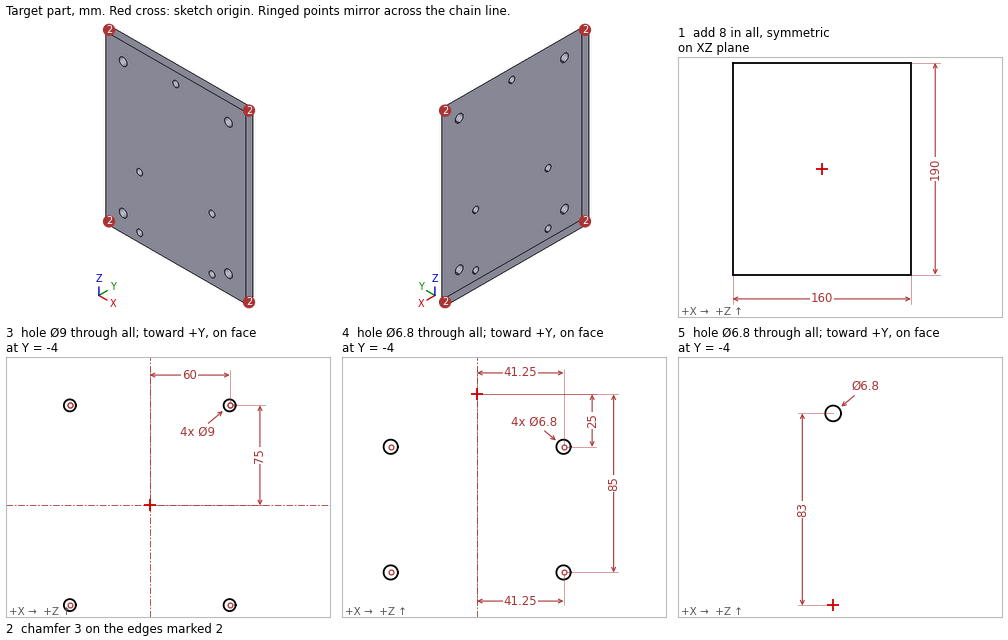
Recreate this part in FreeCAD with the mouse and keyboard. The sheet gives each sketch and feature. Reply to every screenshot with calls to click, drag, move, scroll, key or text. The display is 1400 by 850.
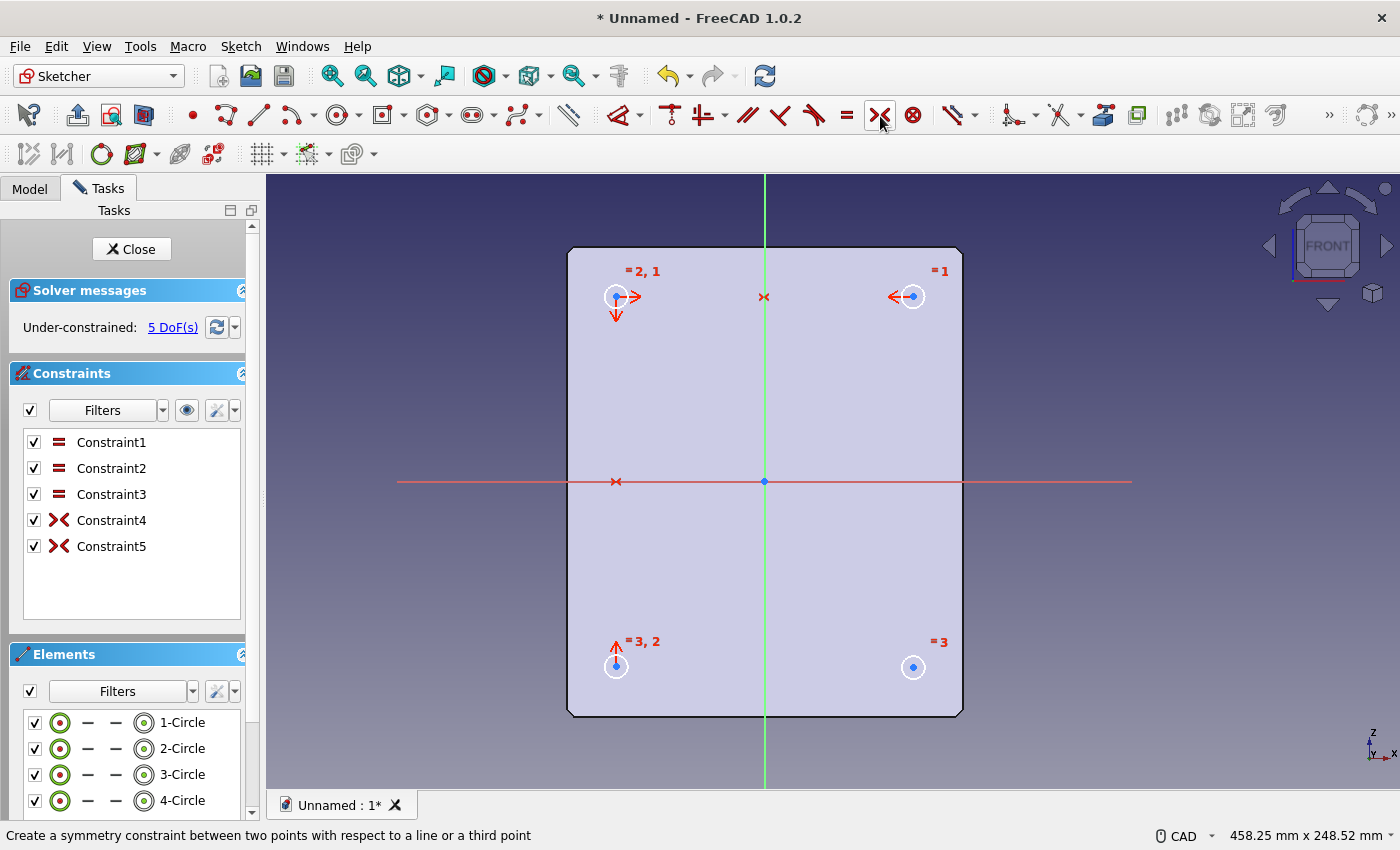
click(913, 297)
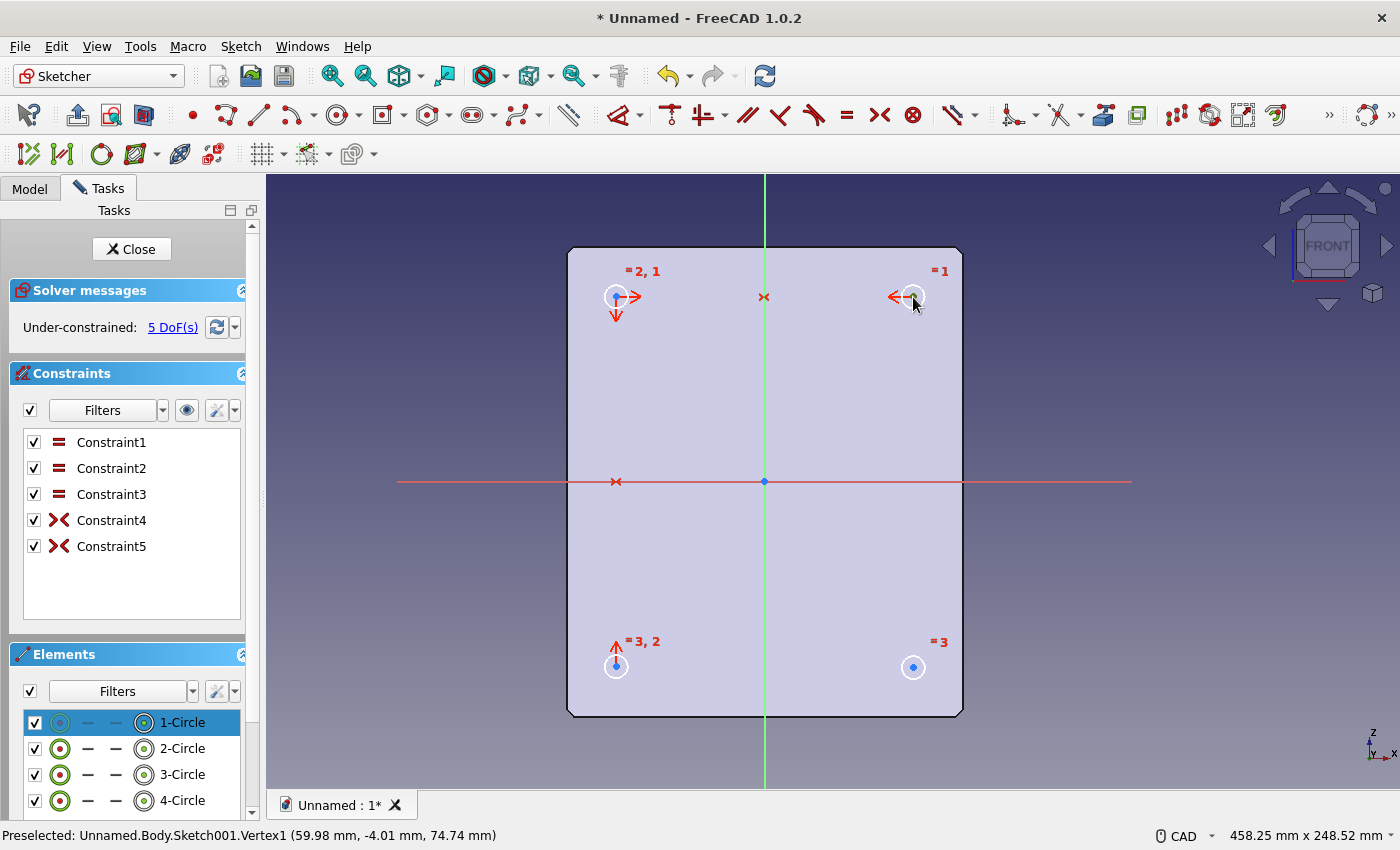
click(913, 668)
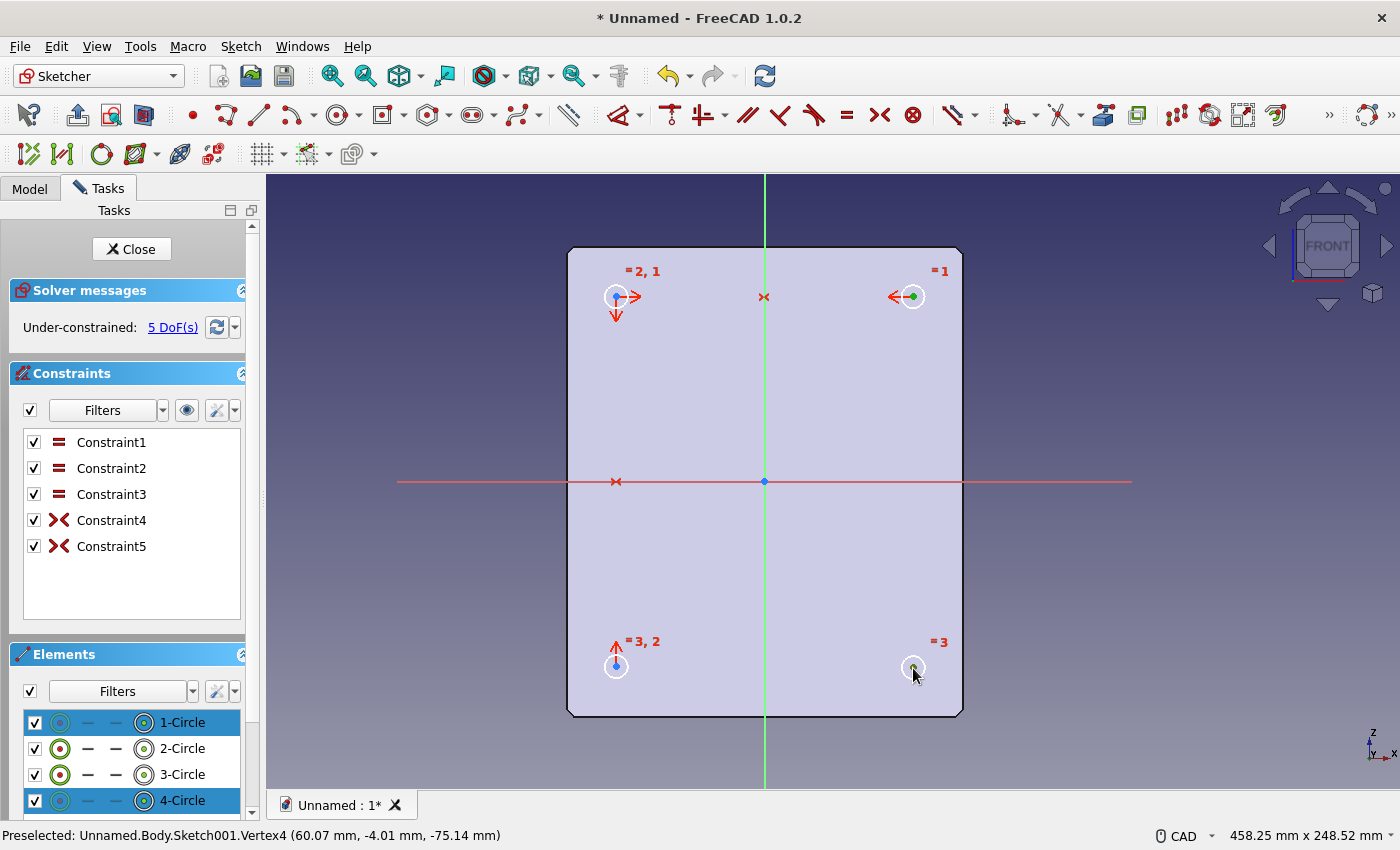
click(428, 482)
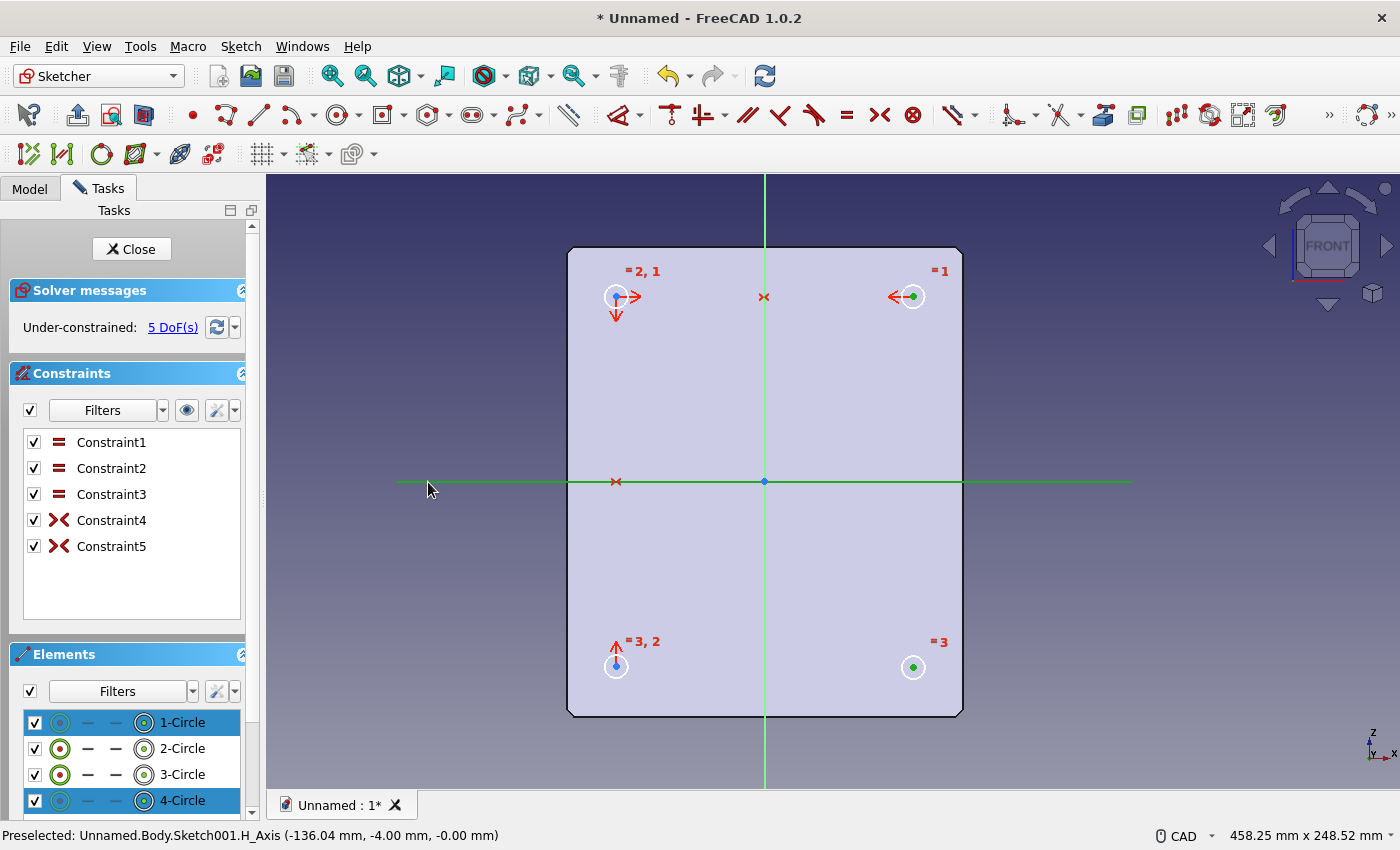
key(s)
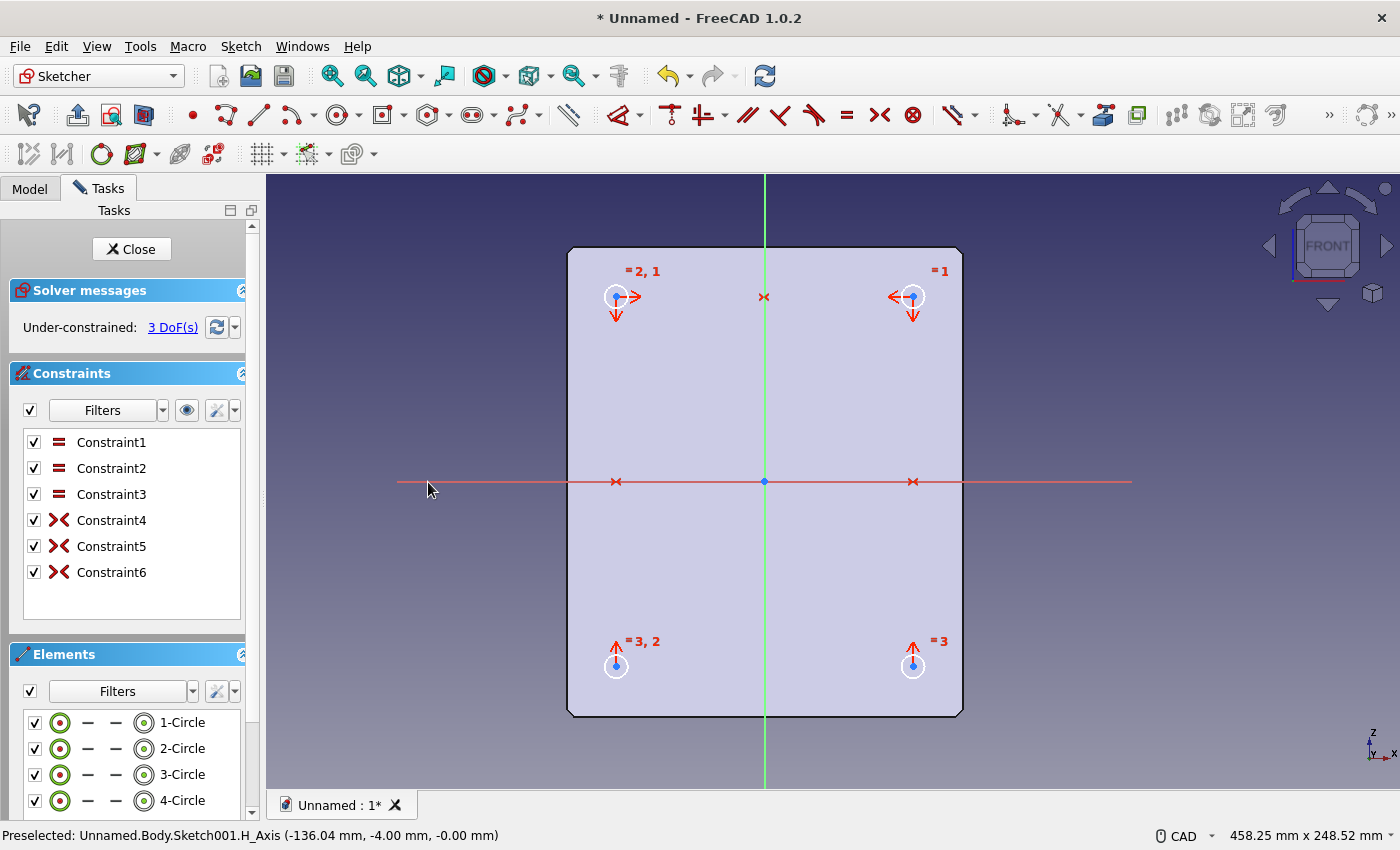
click(618, 116)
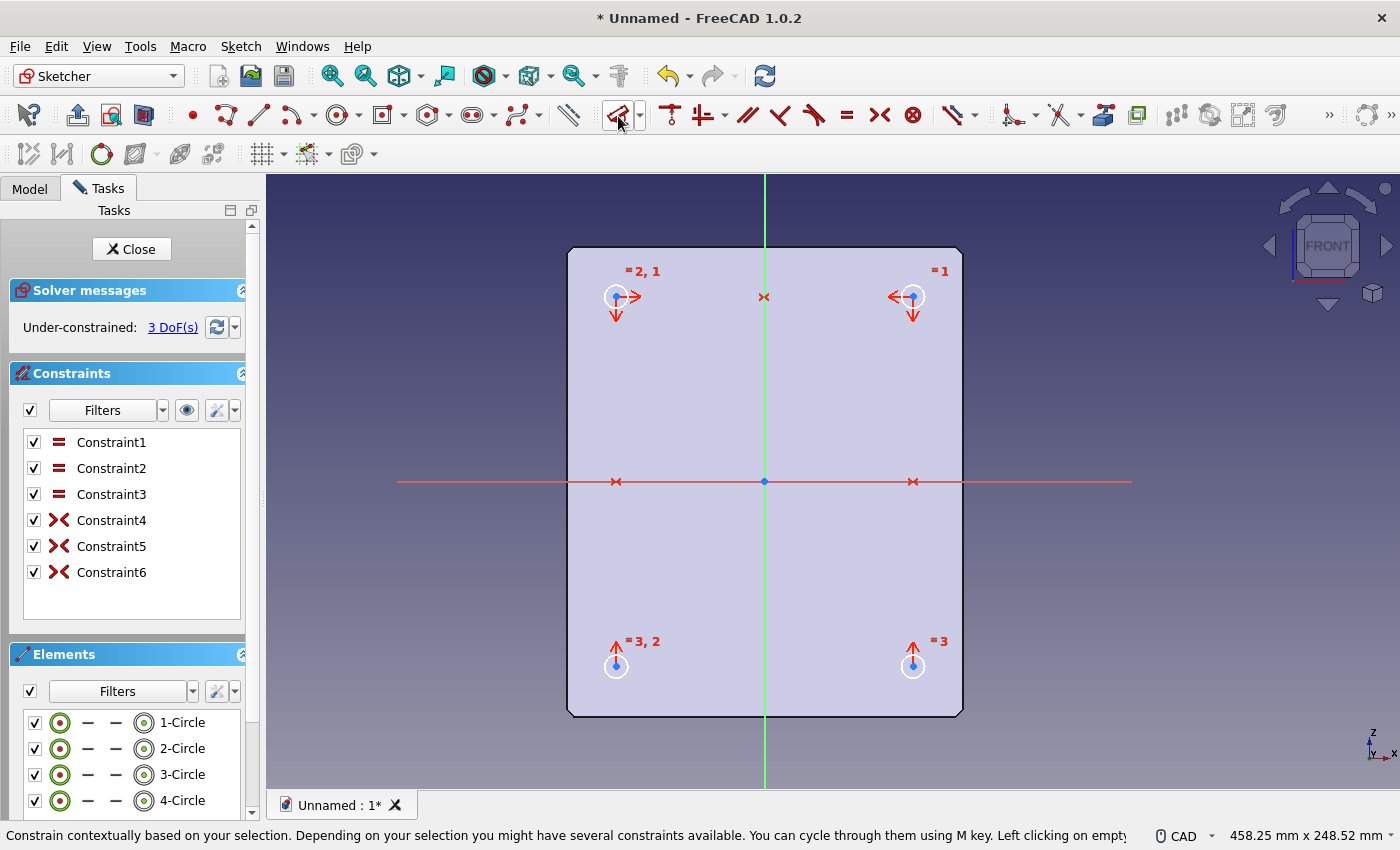
scroll(921, 289, up, 3)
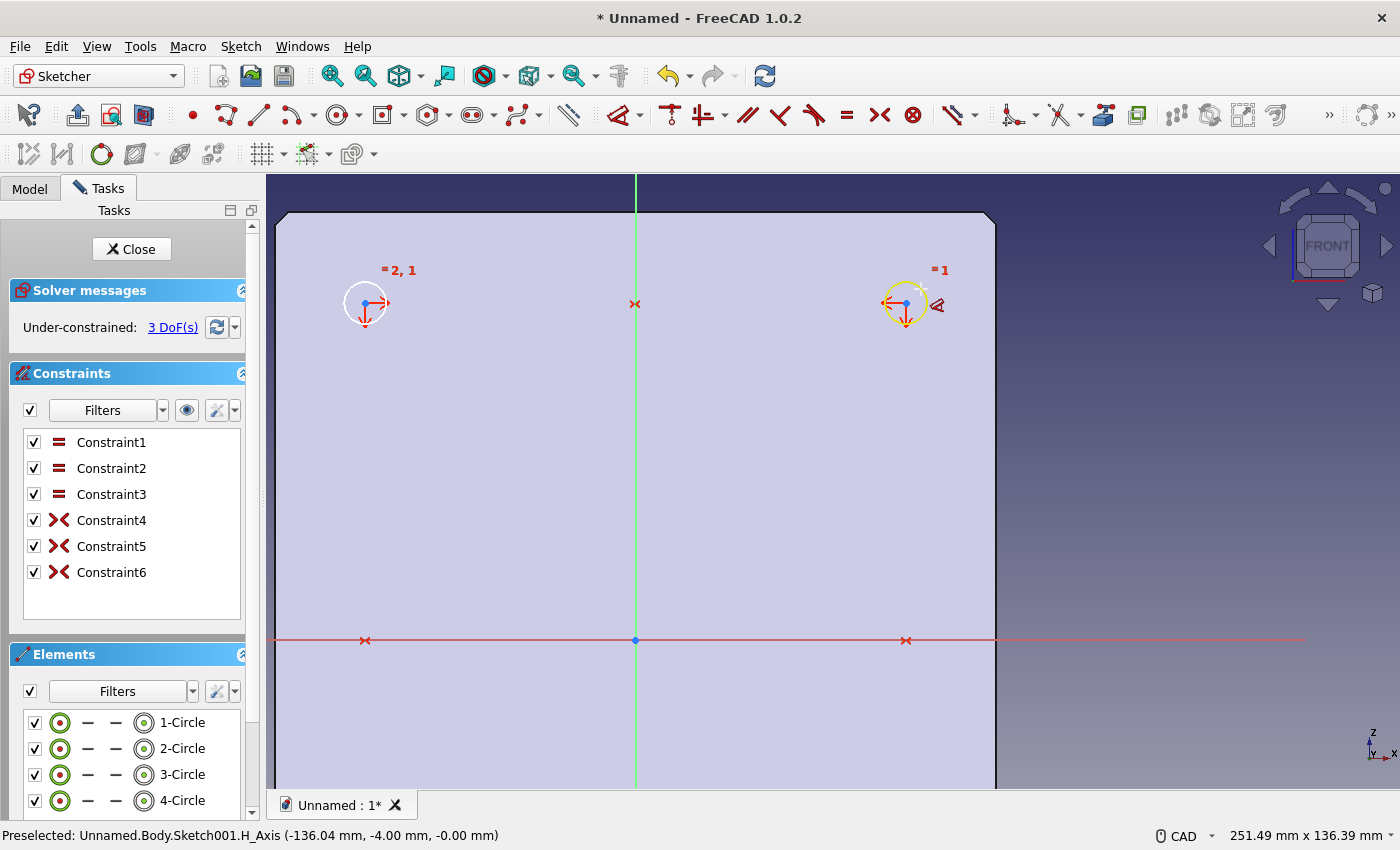
click(921, 288)
click(944, 265)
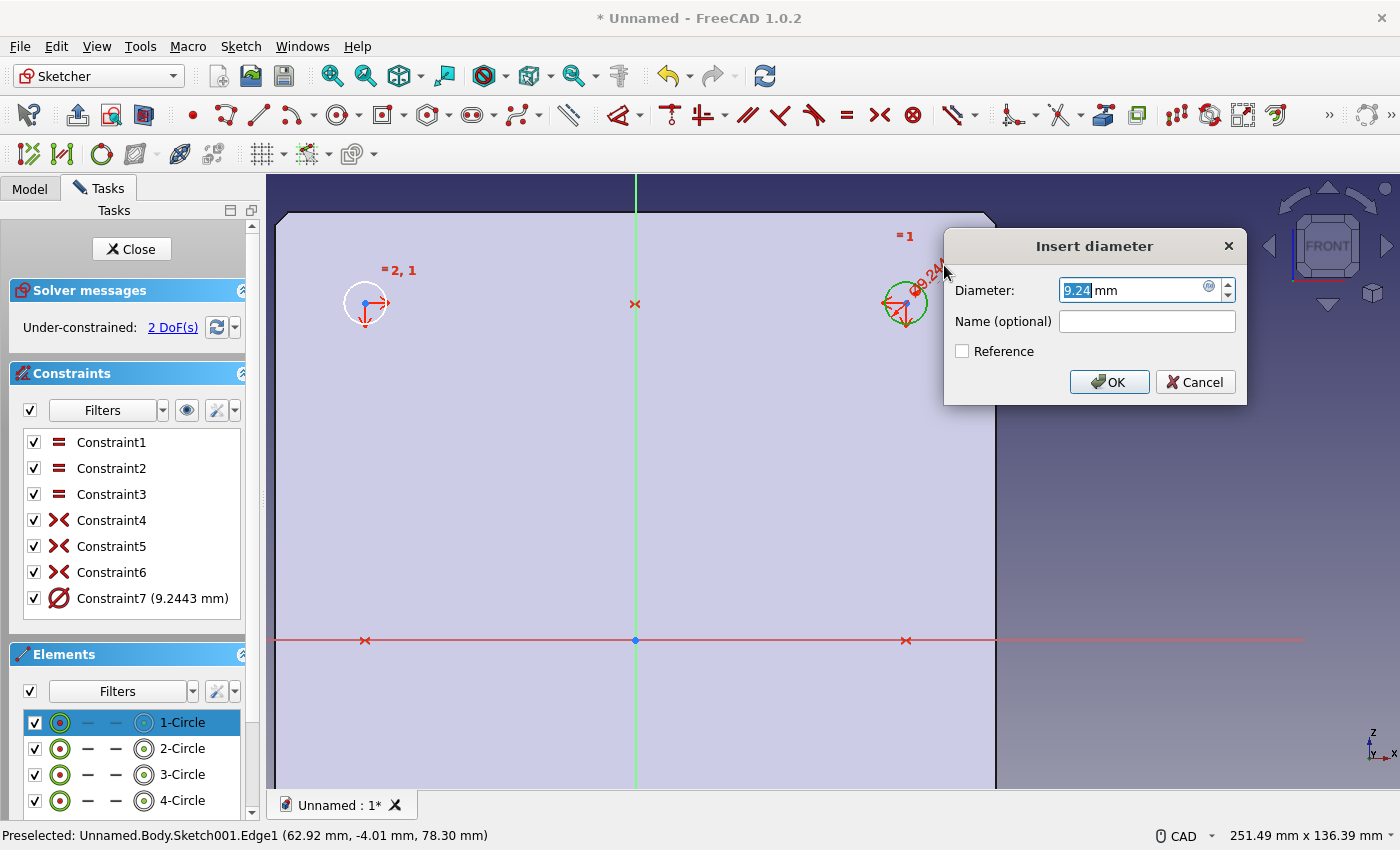
text(9)
key(Return)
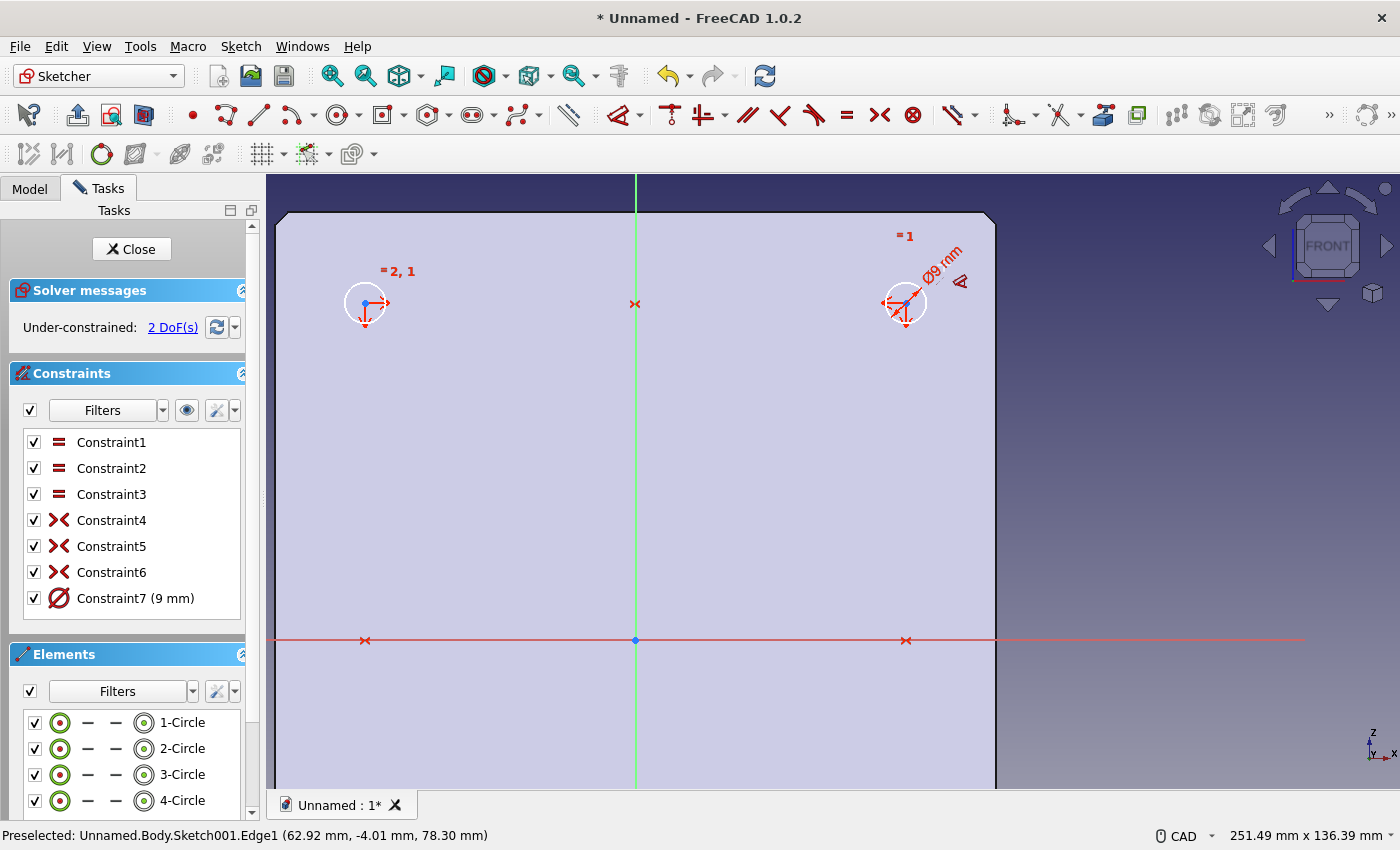
click(906, 303)
click(771, 269)